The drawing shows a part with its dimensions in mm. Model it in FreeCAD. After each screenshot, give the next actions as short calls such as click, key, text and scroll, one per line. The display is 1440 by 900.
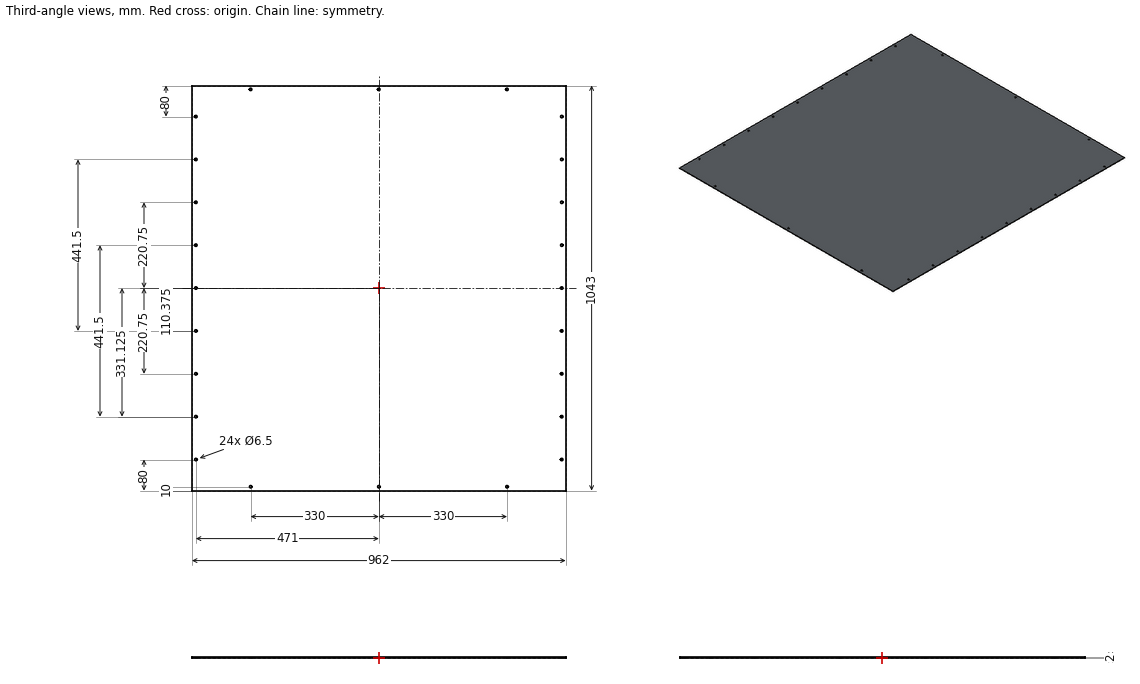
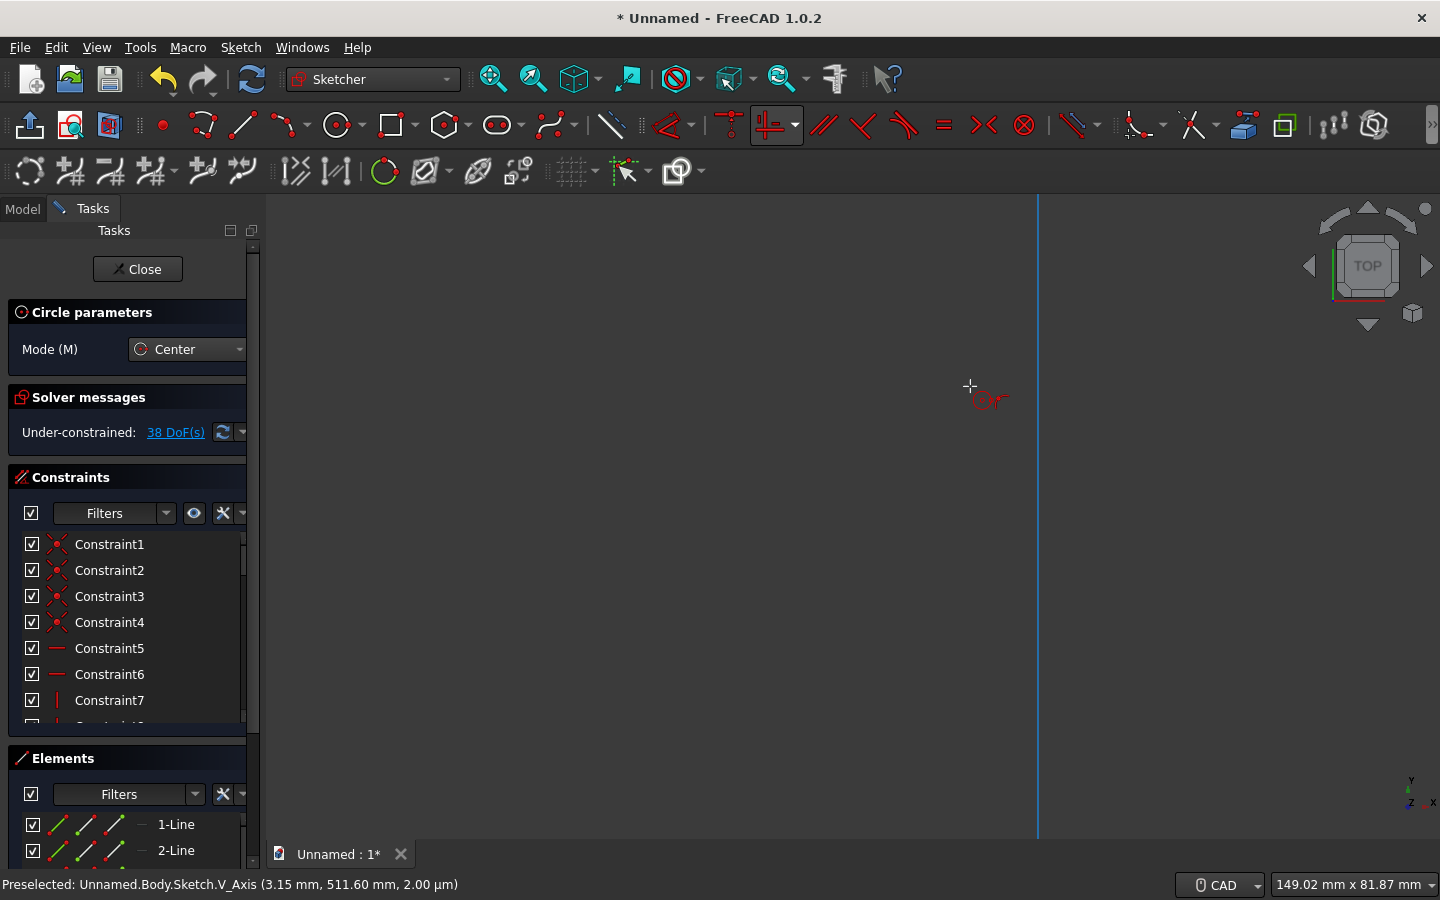
scroll(970, 387, down, 15)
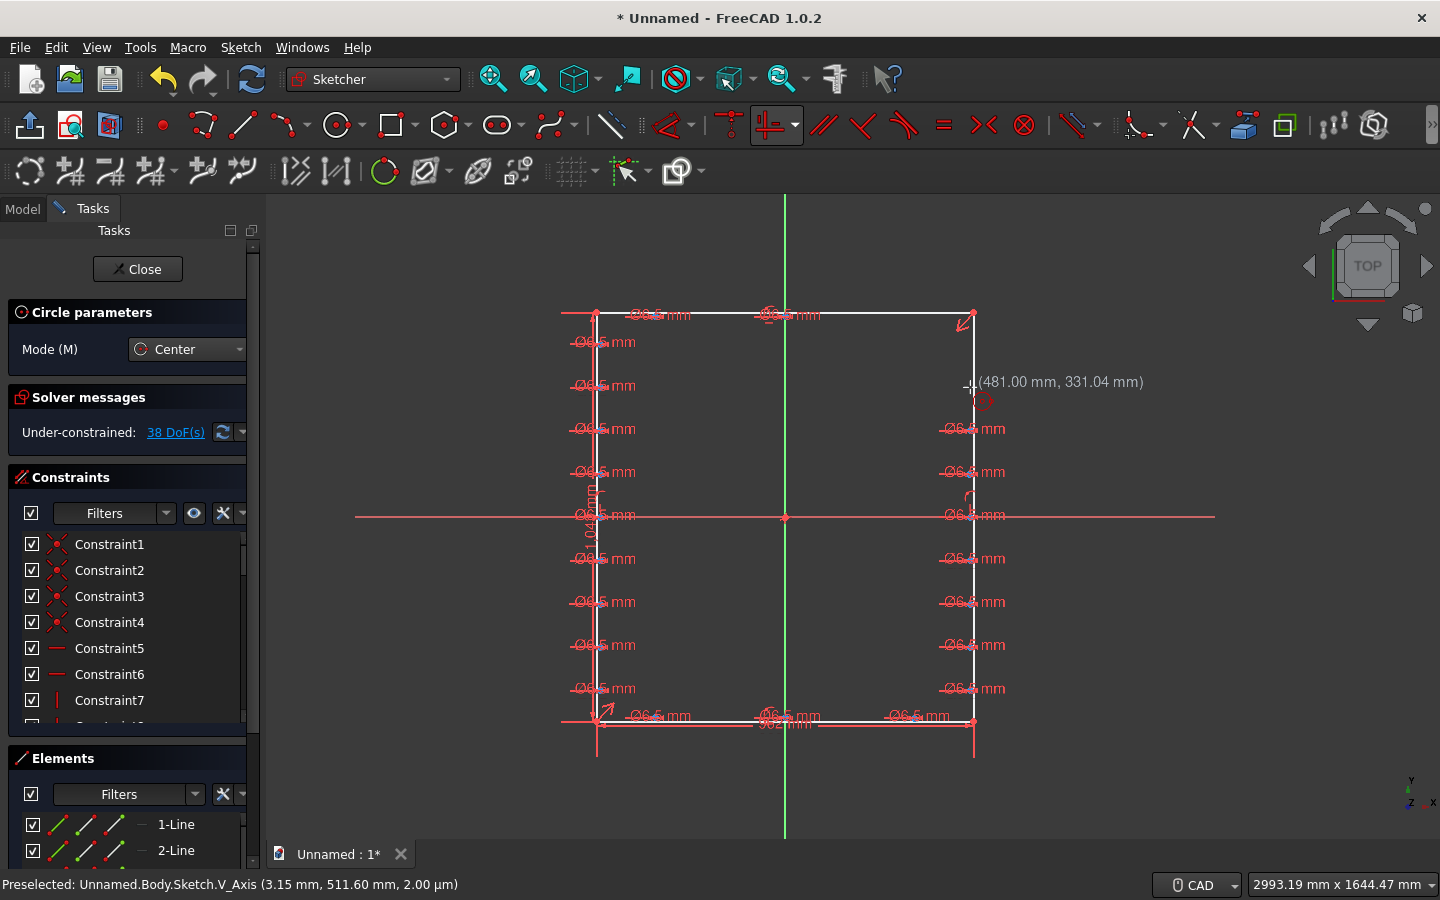
scroll(970, 387, up, 7)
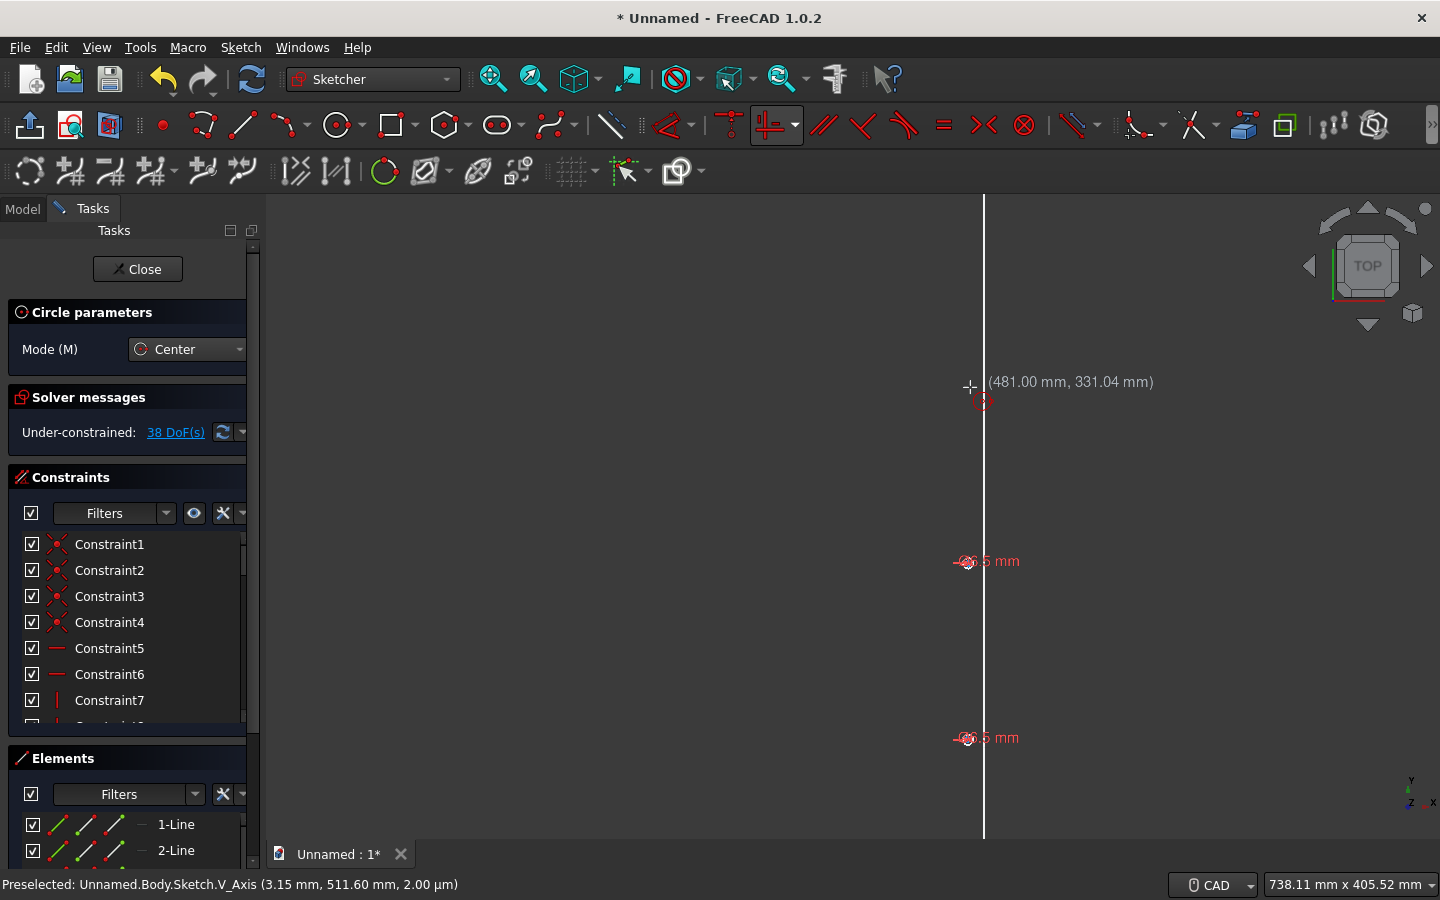
click(968, 387)
move(965, 384)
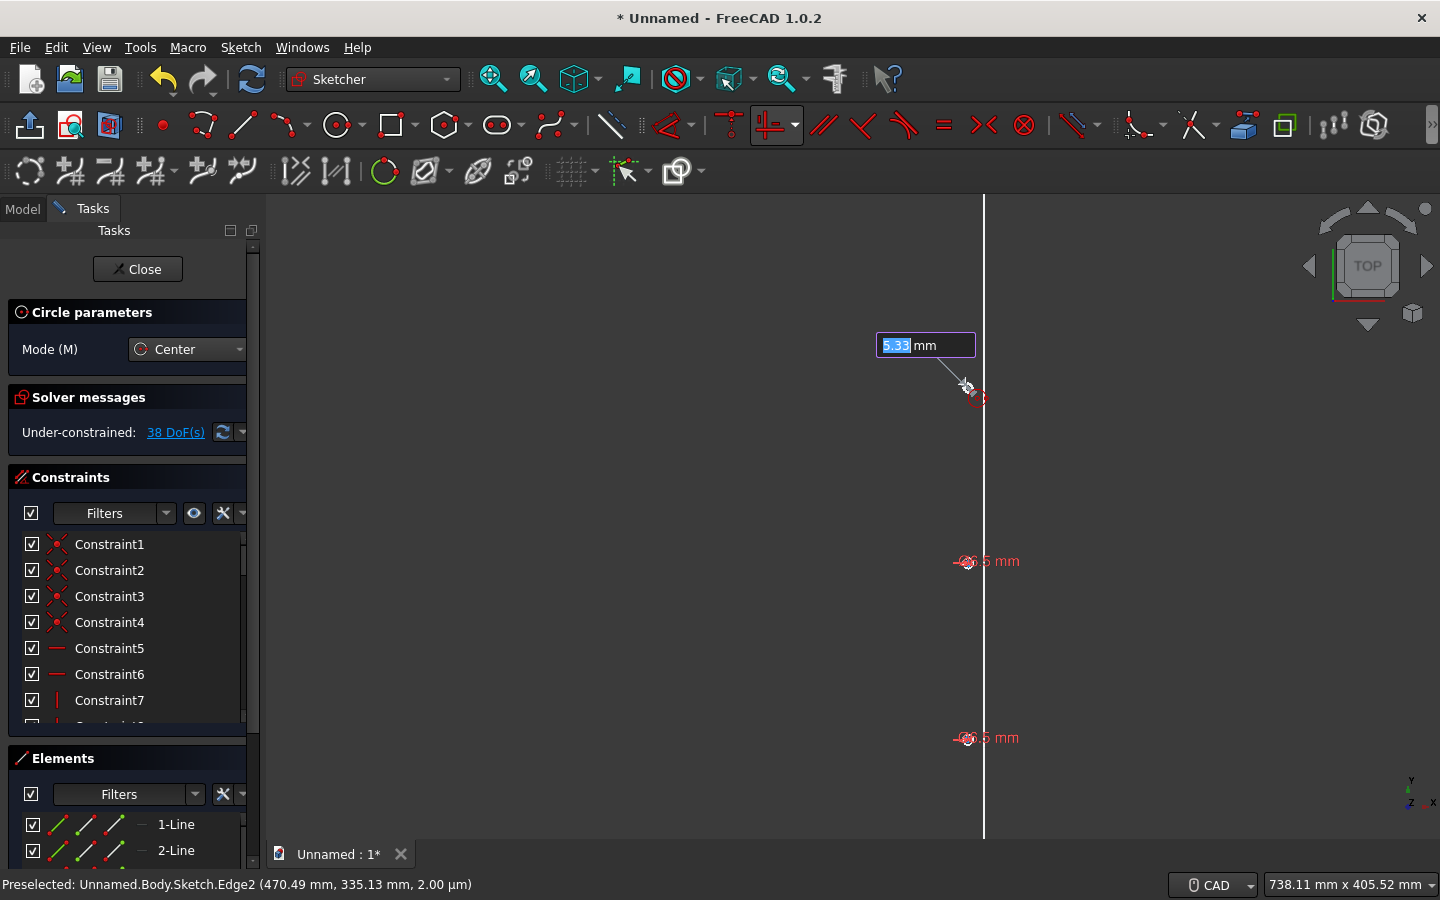
text(6.5)
key(Return)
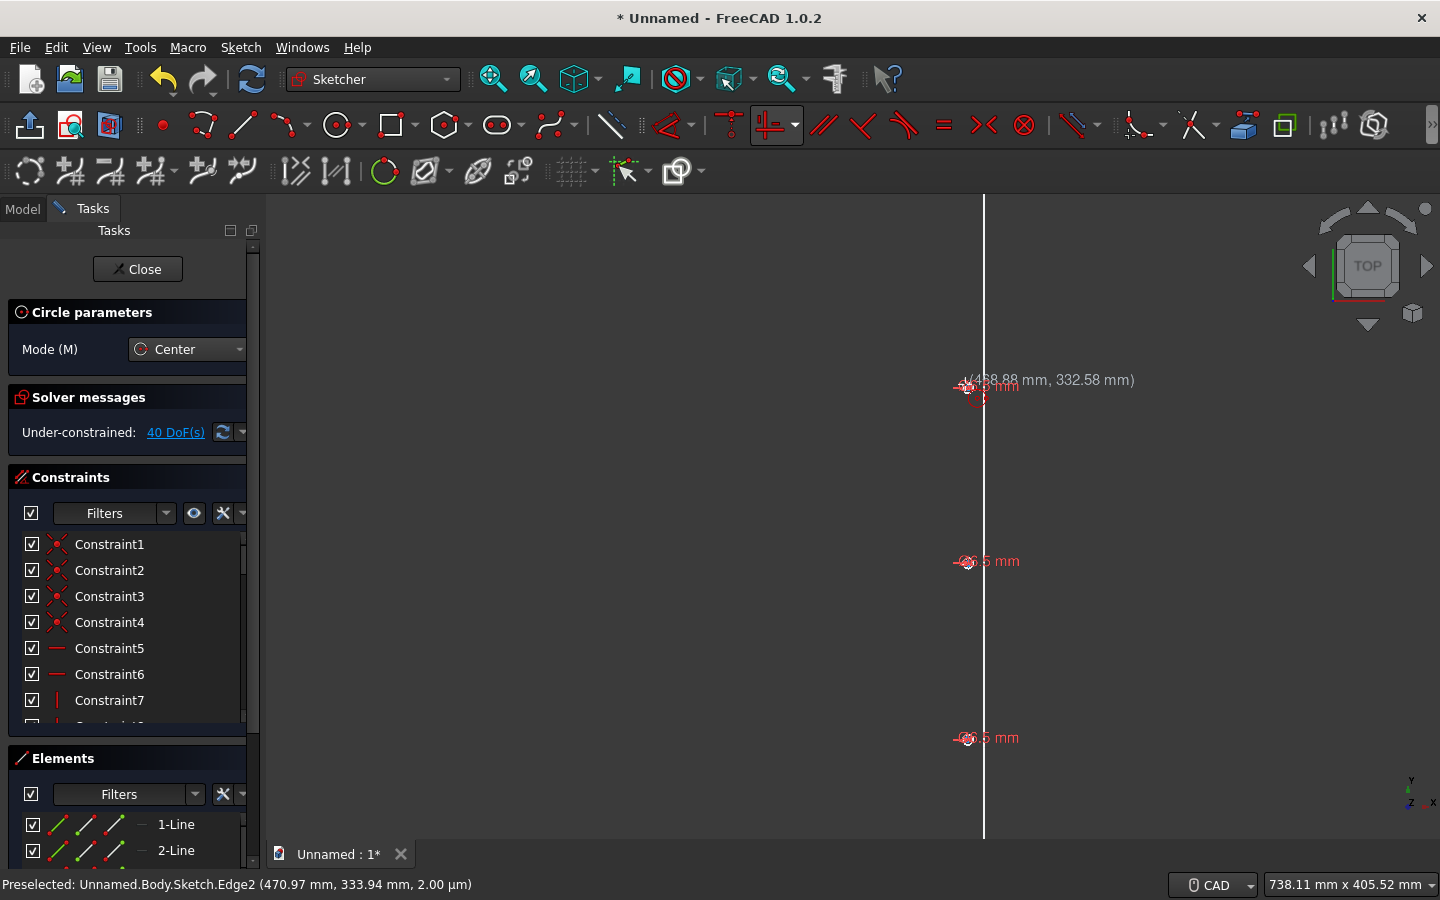
scroll(970, 386, down, 7)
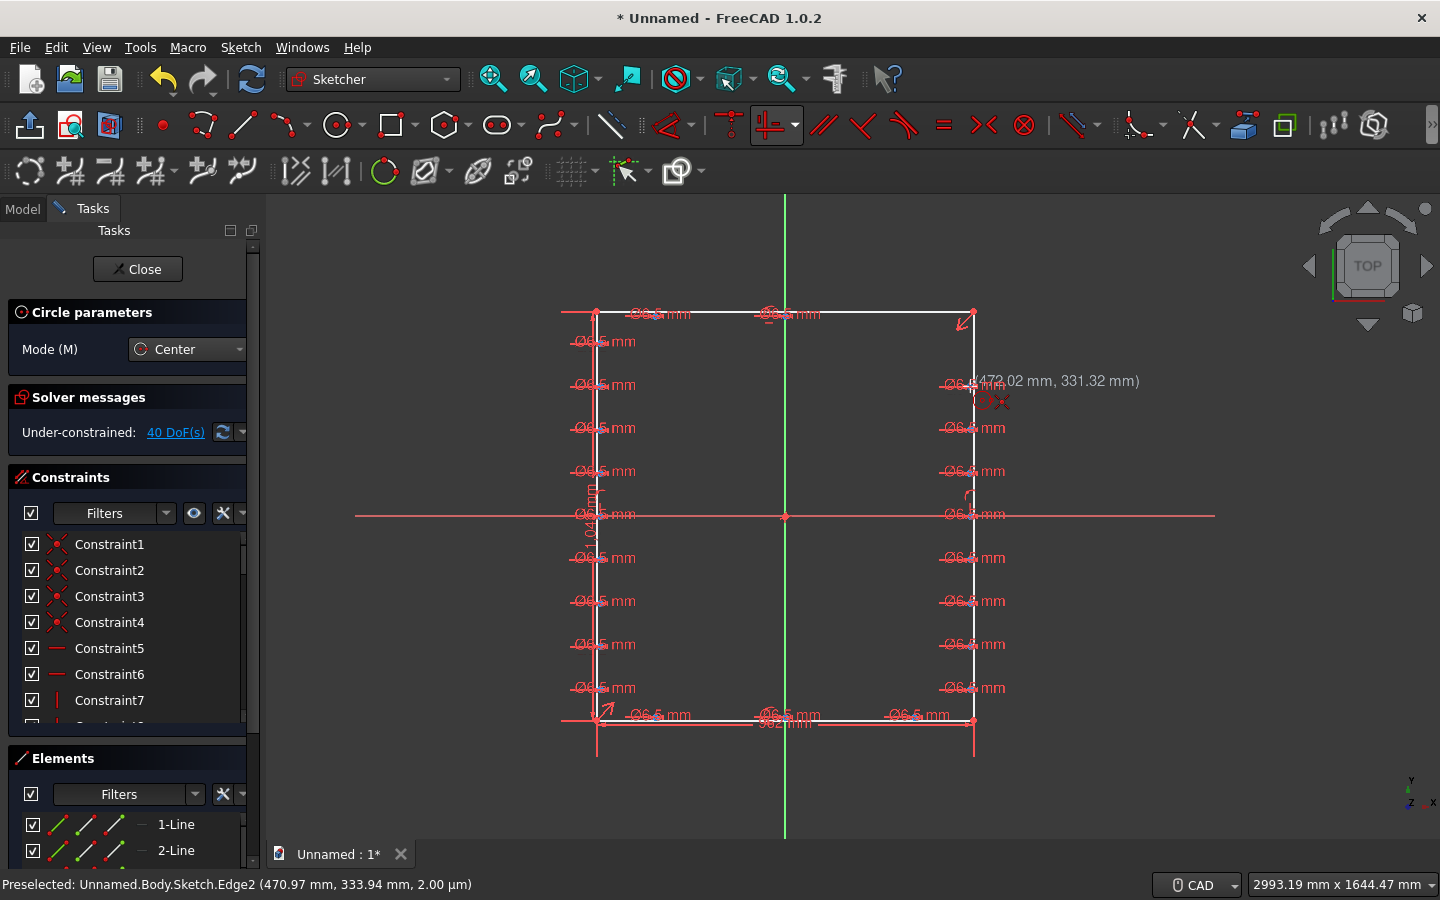
scroll(915, 316, up, 15)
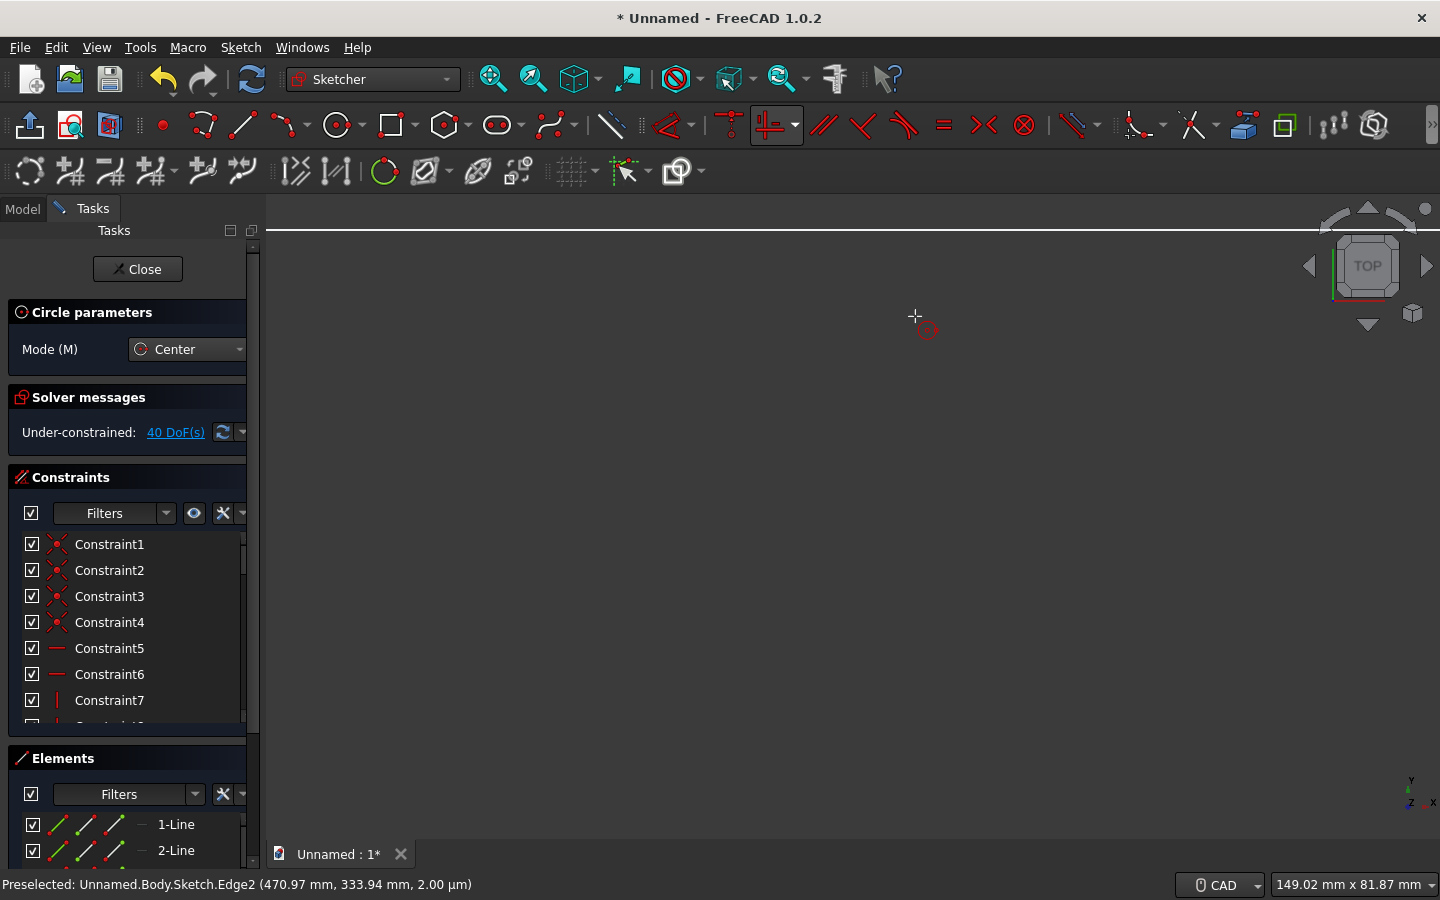
scroll(915, 316, down, 15)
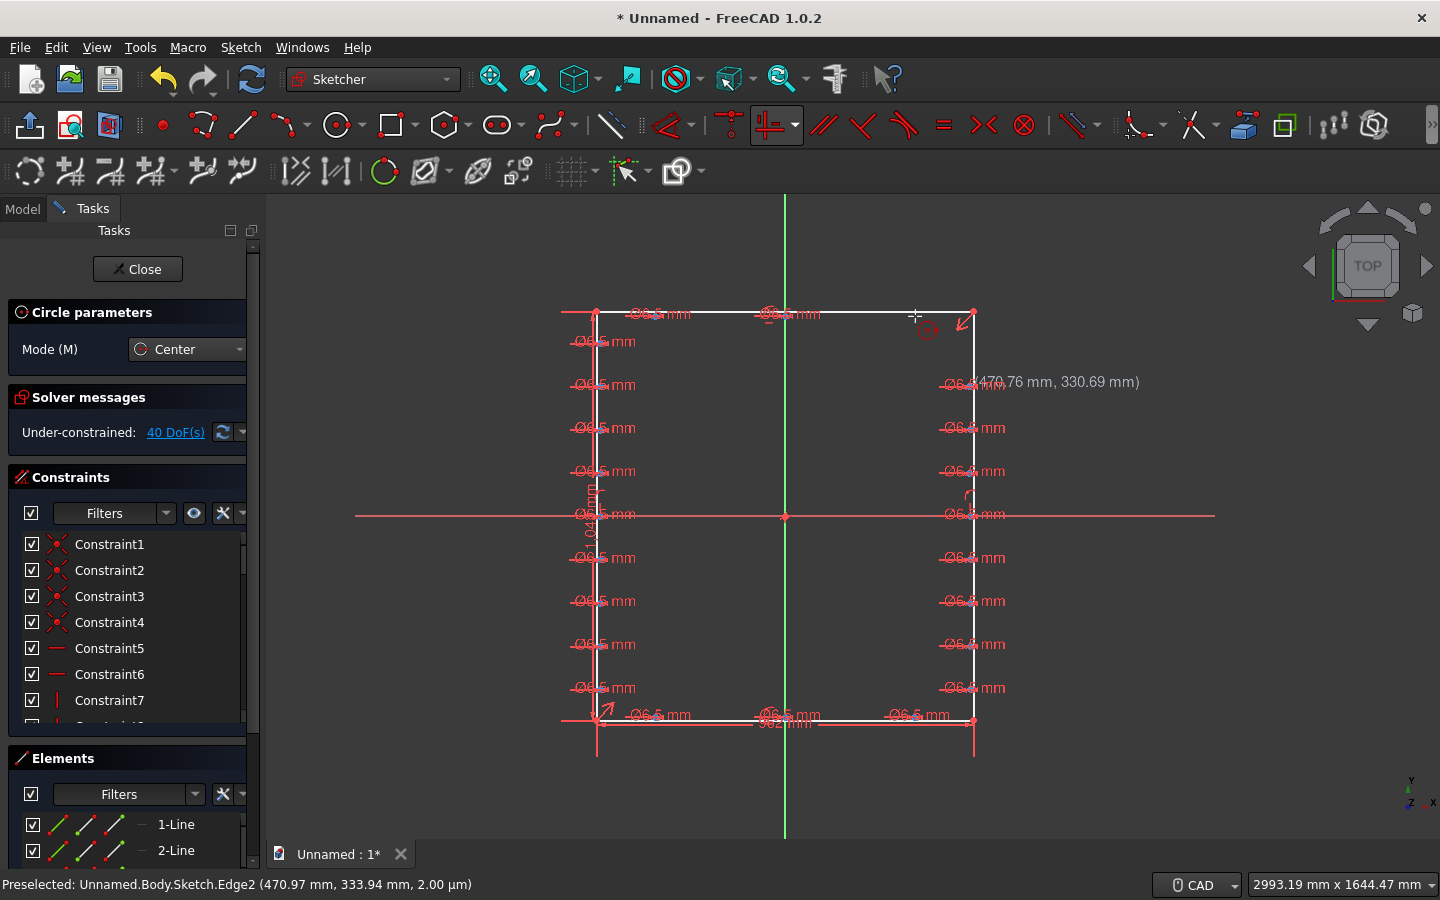
scroll(915, 316, up, 7)